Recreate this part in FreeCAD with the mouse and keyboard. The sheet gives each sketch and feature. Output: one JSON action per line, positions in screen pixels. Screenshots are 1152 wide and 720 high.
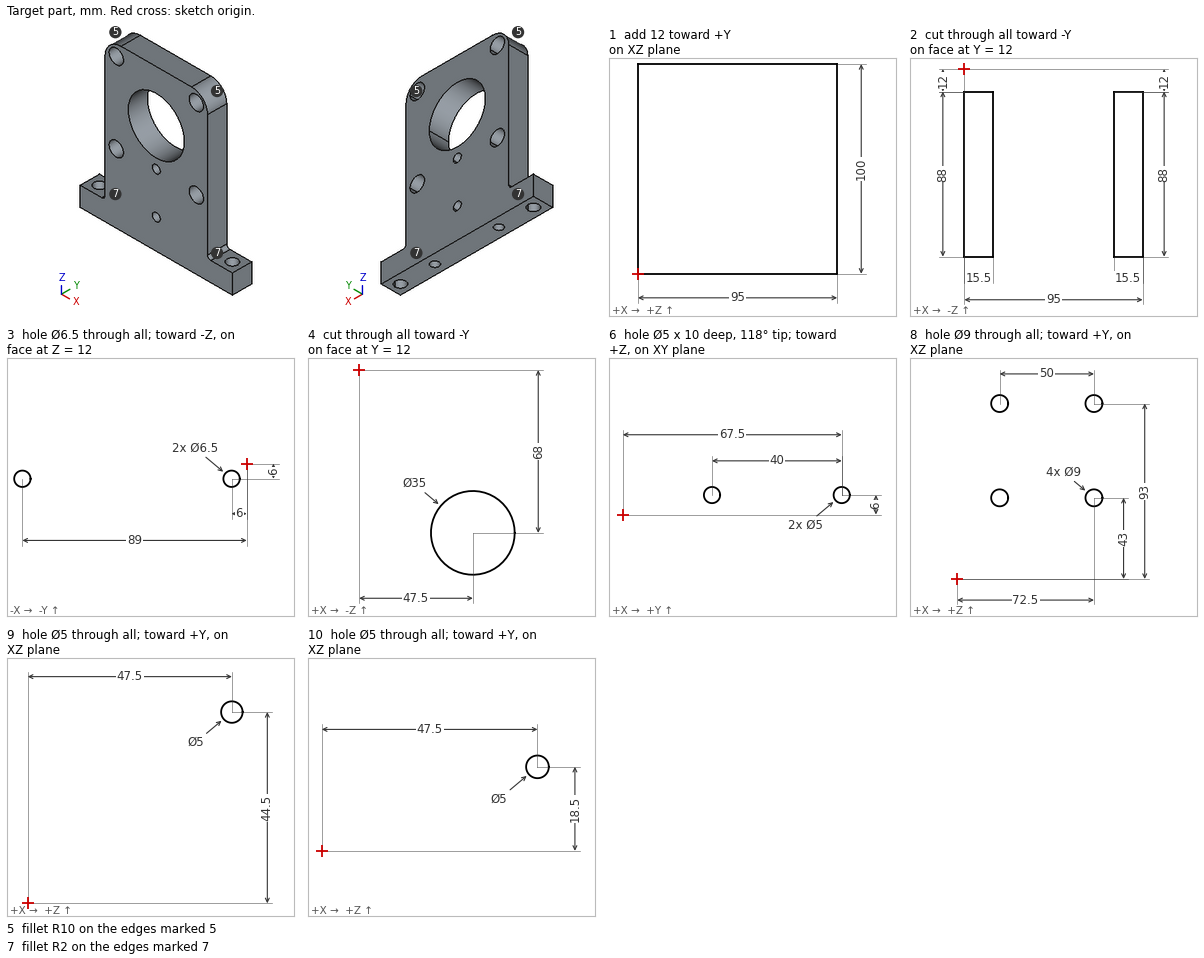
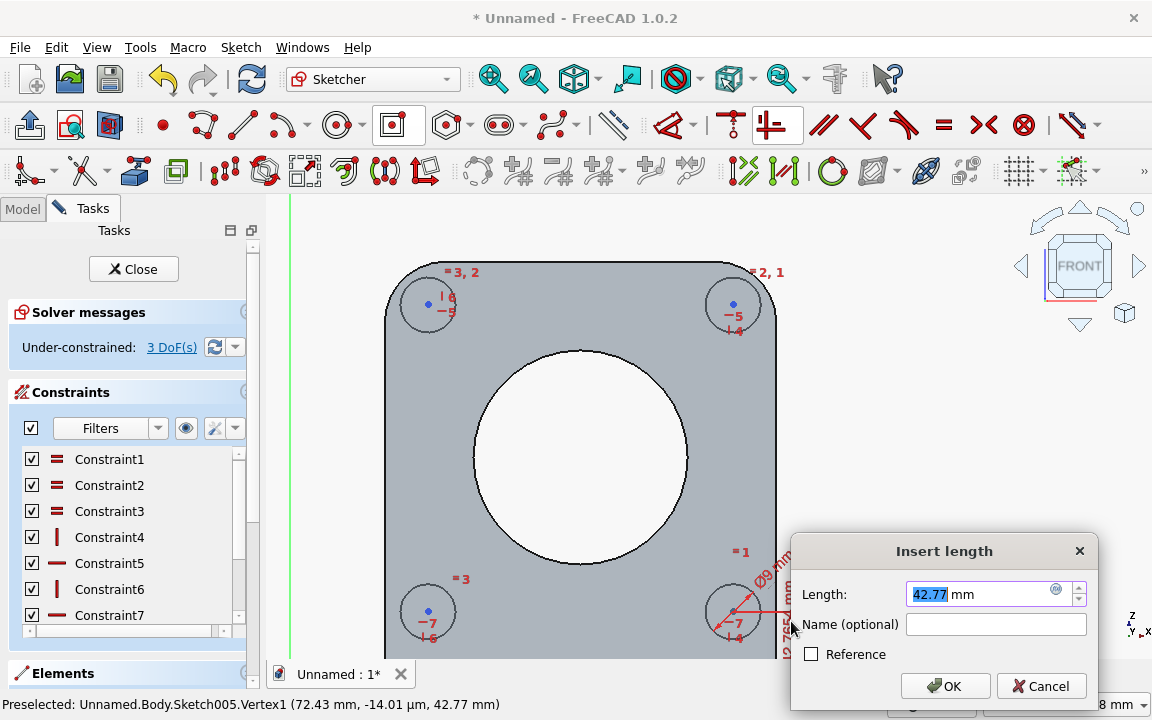
{"action": "type", "text": "43"}
{"action": "key", "text": "Return"}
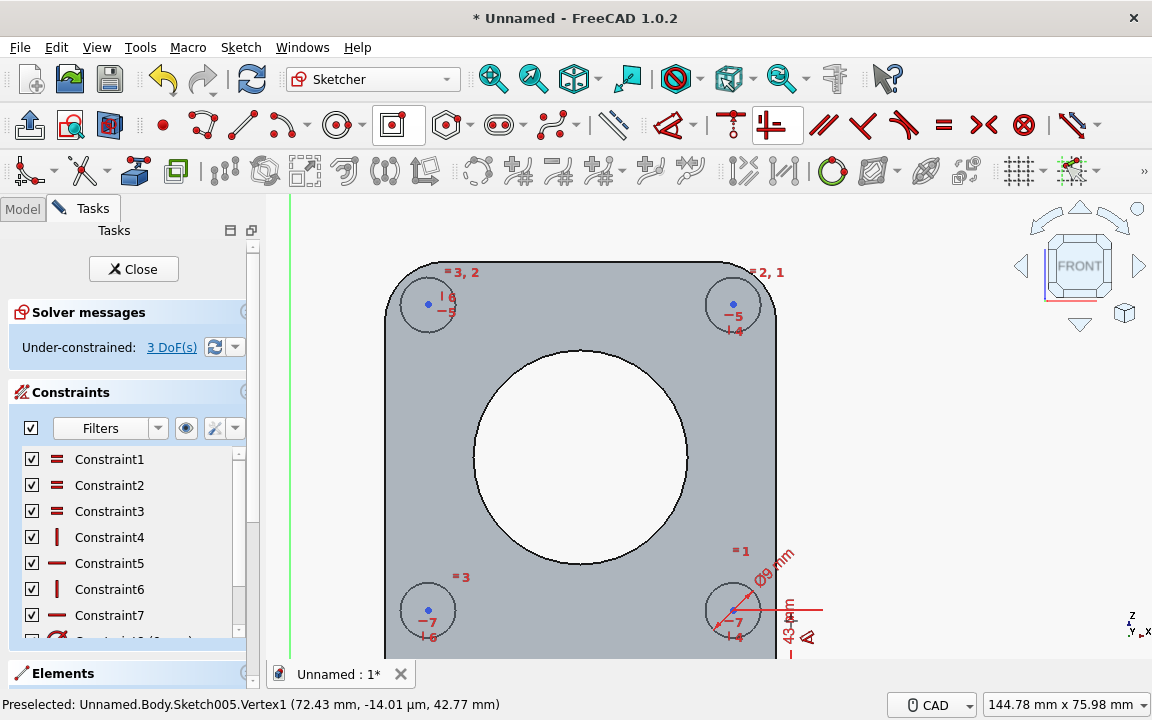
{"action": "left_click", "coordinate": [733, 305]}
{"action": "left_click", "coordinate": [767, 468]}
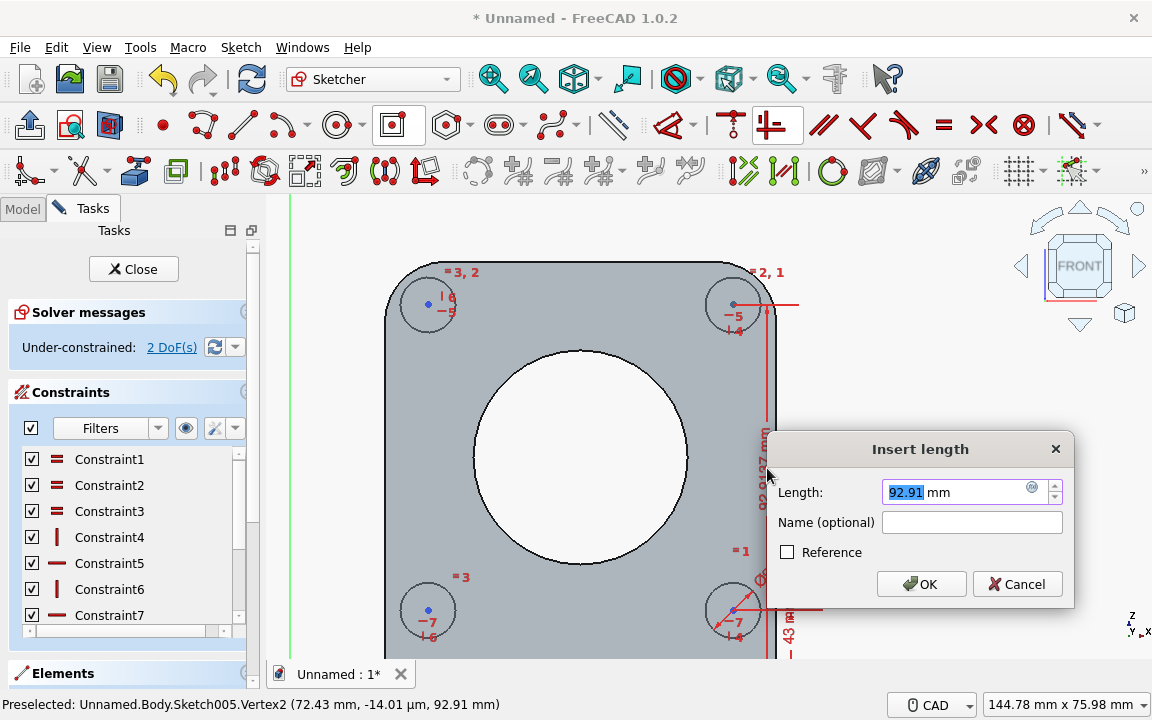
{"action": "type", "text": "93"}
{"action": "key", "text": "Return"}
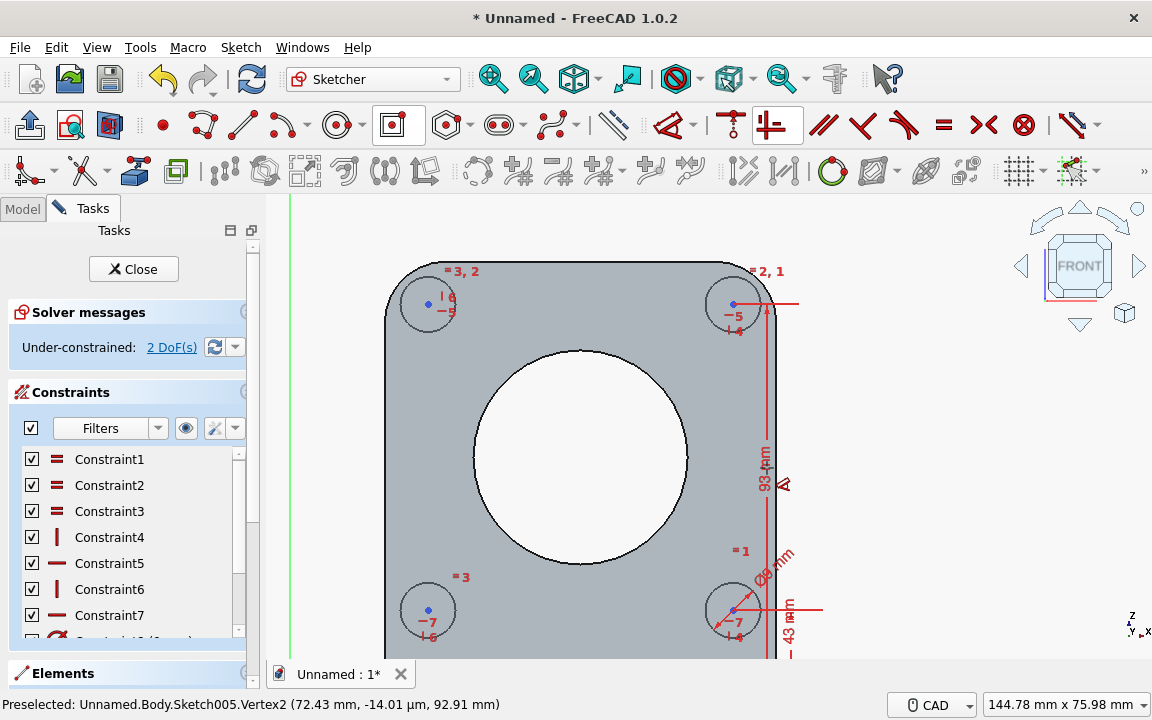
{"action": "left_click", "coordinate": [733, 304]}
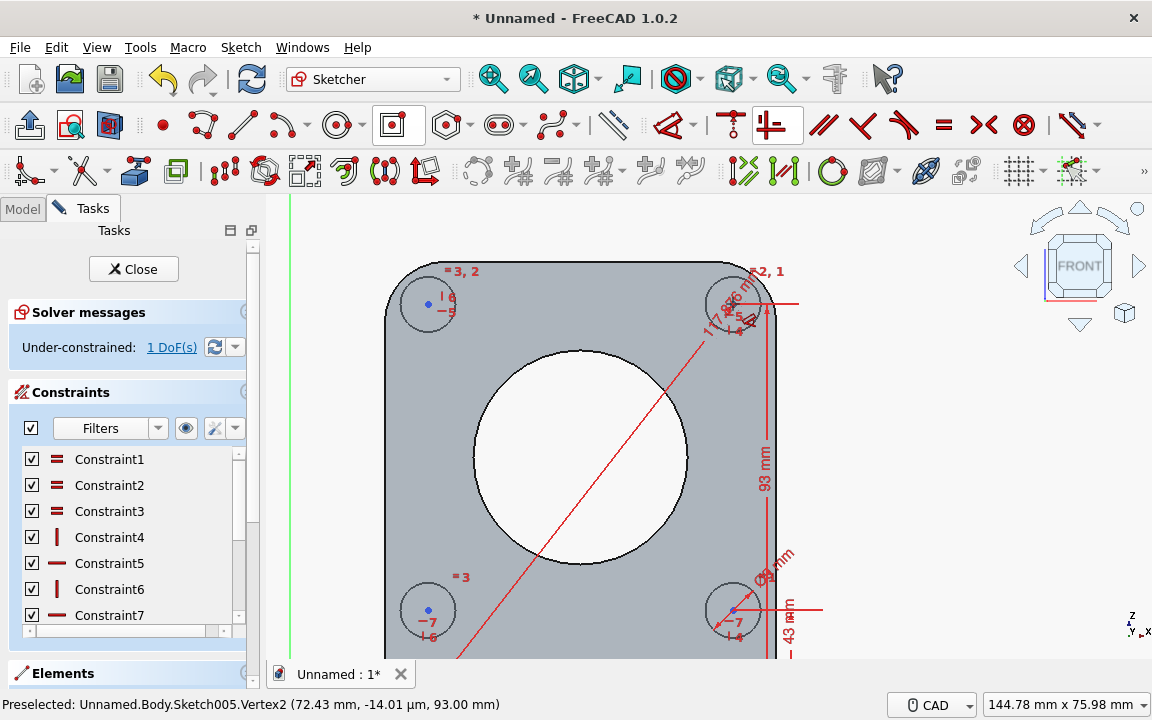
{"action": "left_click", "coordinate": [428, 304]}
{"action": "left_click", "coordinate": [581, 270]}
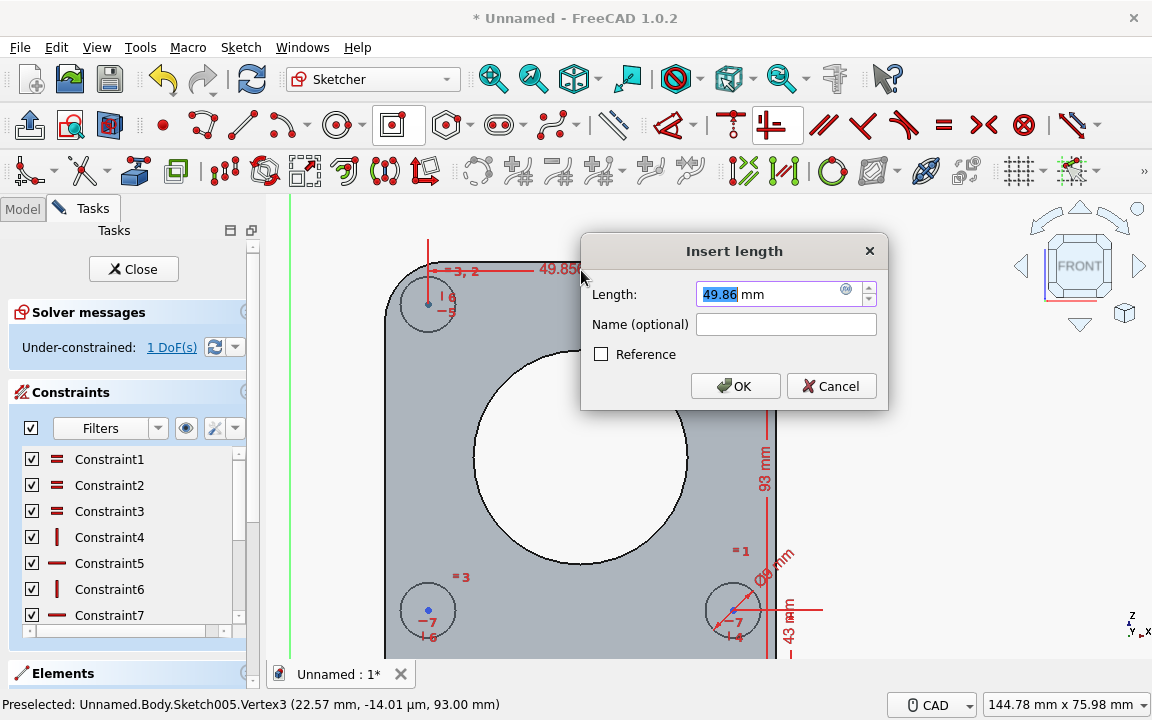
{"action": "type", "text": "50"}
{"action": "key", "text": "Return"}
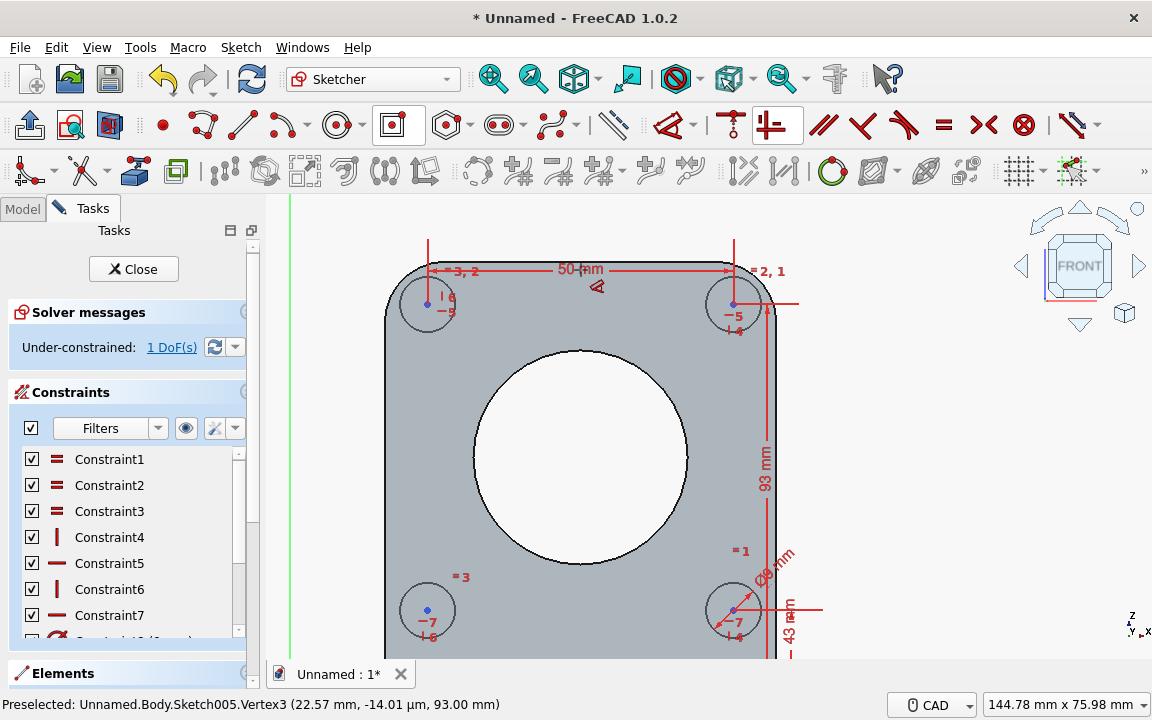
{"action": "left_click", "coordinate": [734, 610]}
{"action": "left_click", "coordinate": [514, 576]}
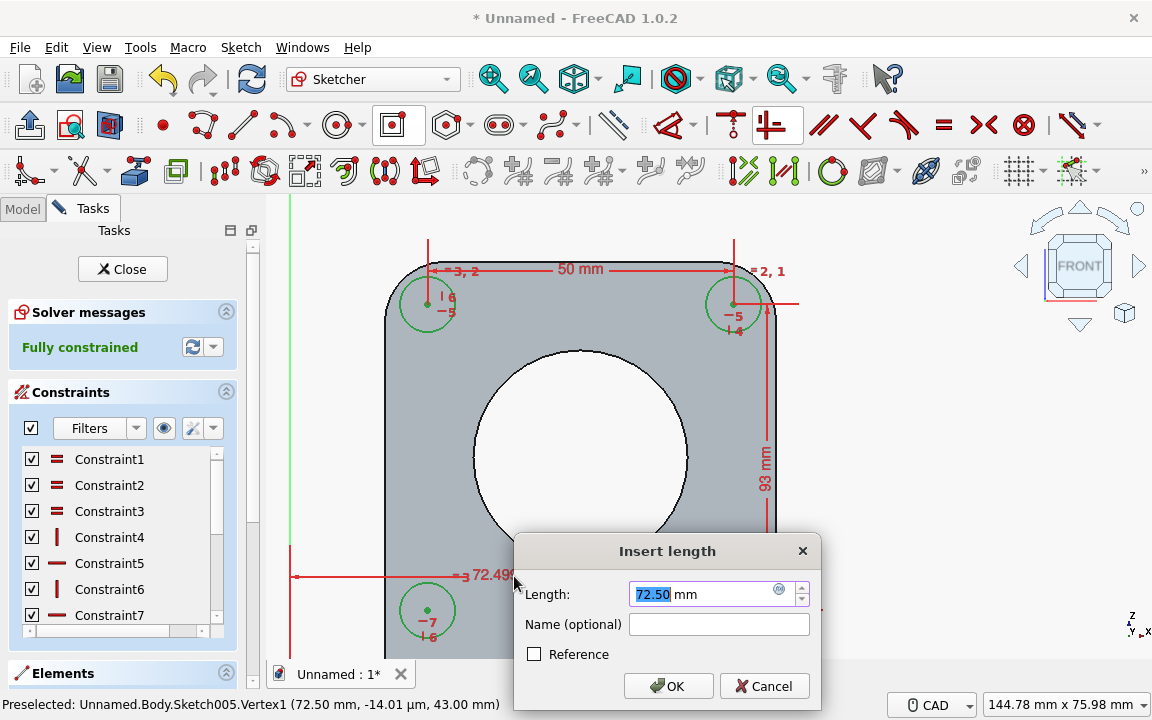
{"action": "type", "text": "72.5"}
{"action": "key", "text": "Return"}
{"action": "key", "text": "Escape"}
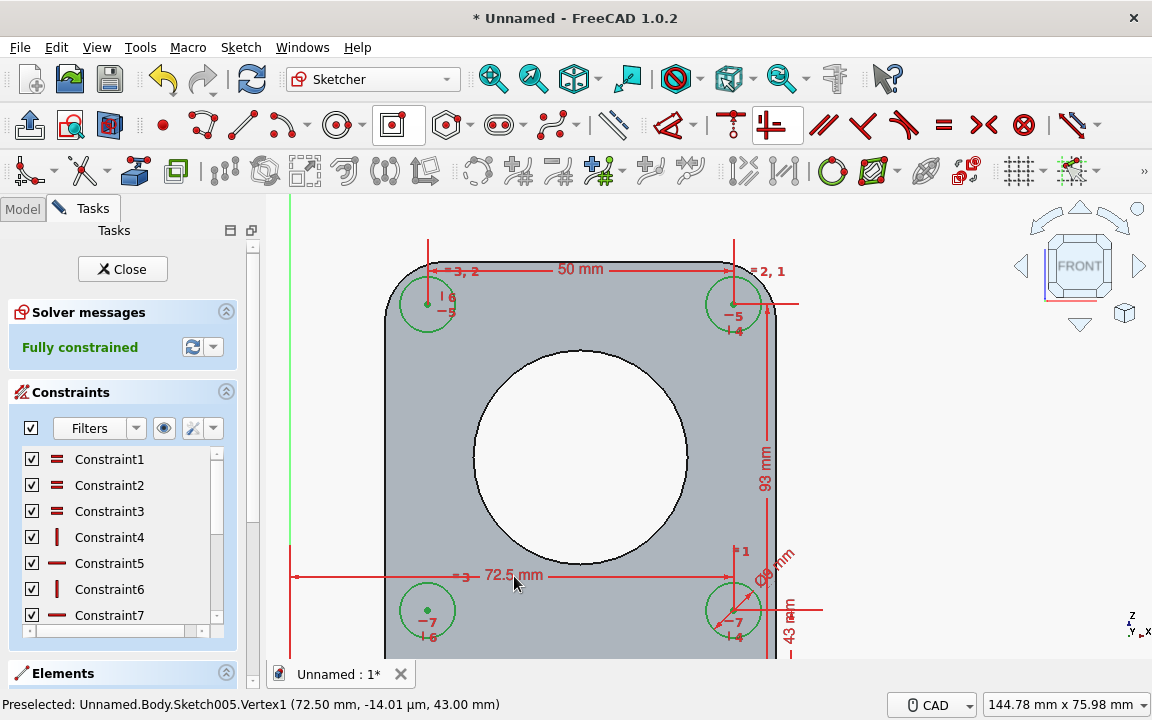
{"action": "left_click", "coordinate": [123, 269]}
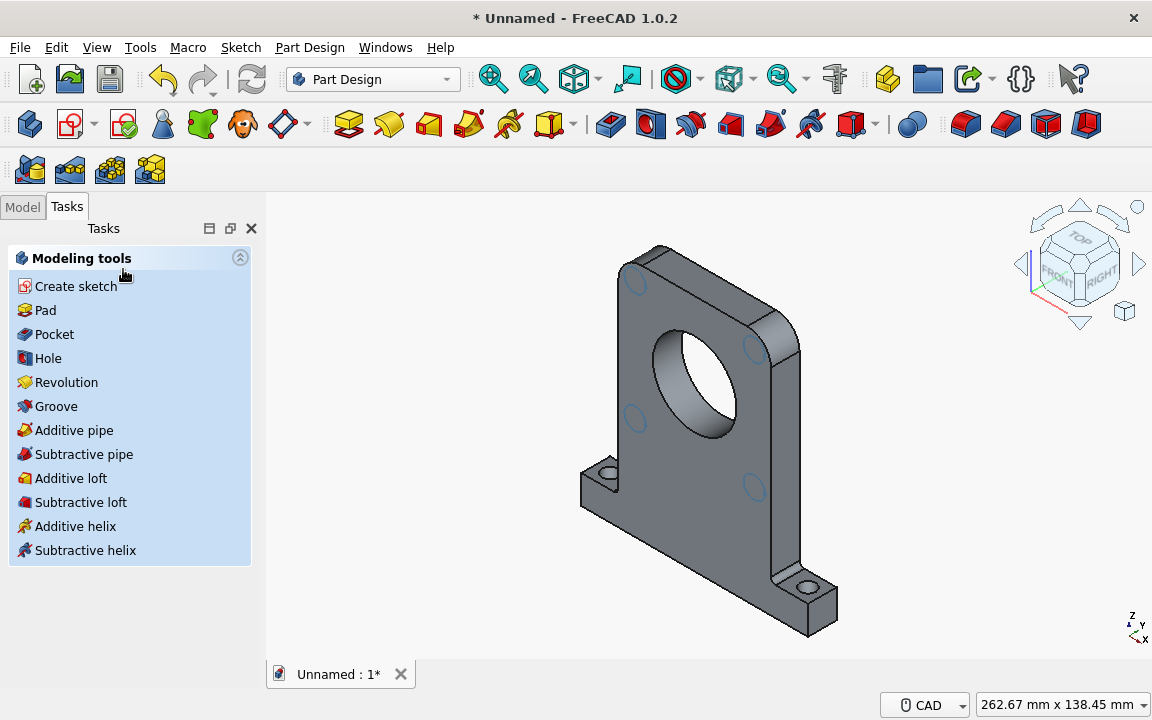
{"action": "left_click", "coordinate": [652, 124]}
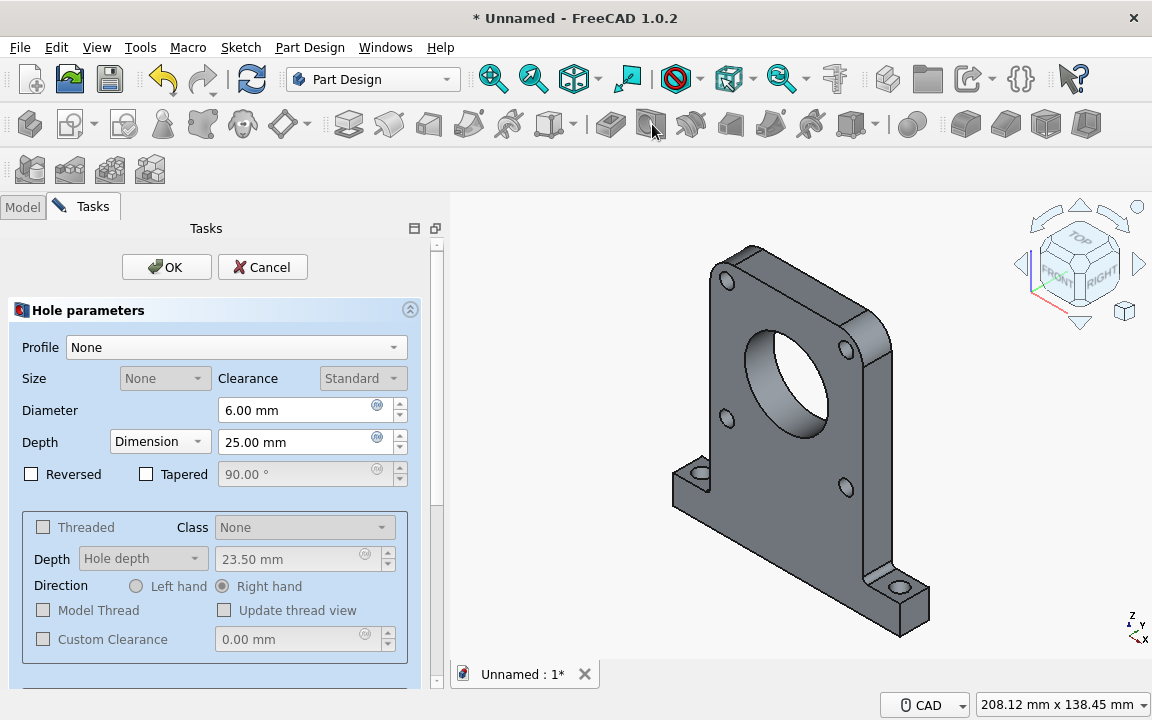
{"action": "triple_click", "coordinate": [305, 410]}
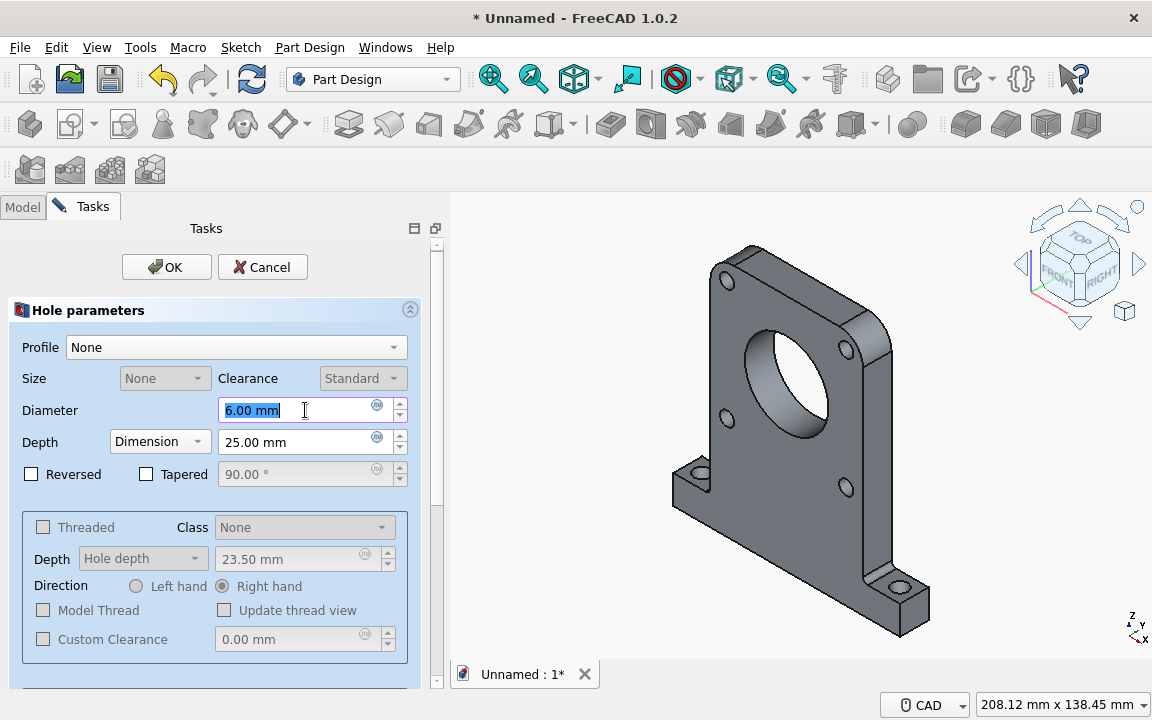
{"action": "type", "text": "9"}
{"action": "key", "text": "Tab"}